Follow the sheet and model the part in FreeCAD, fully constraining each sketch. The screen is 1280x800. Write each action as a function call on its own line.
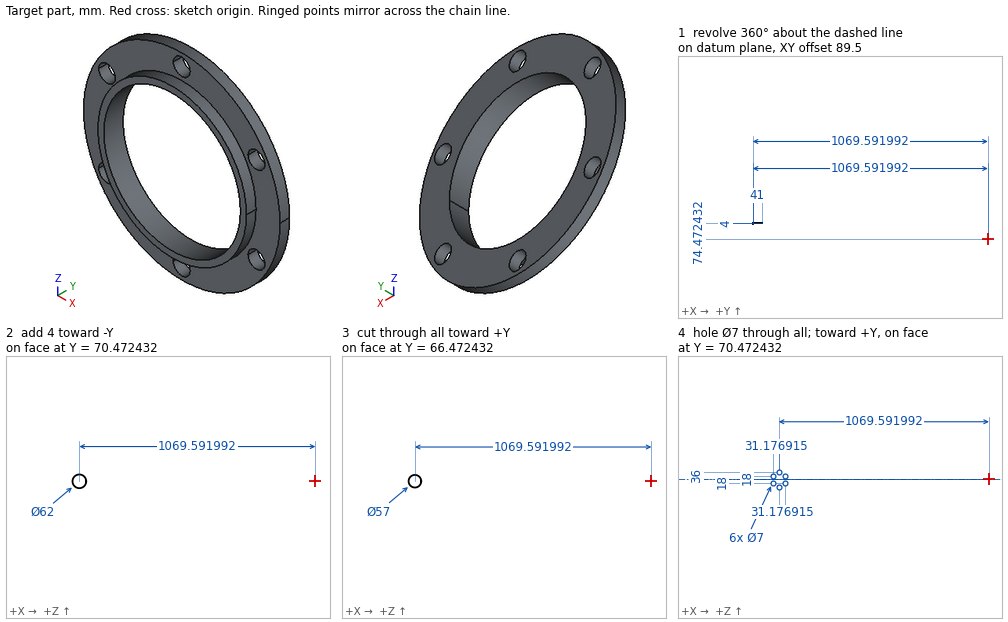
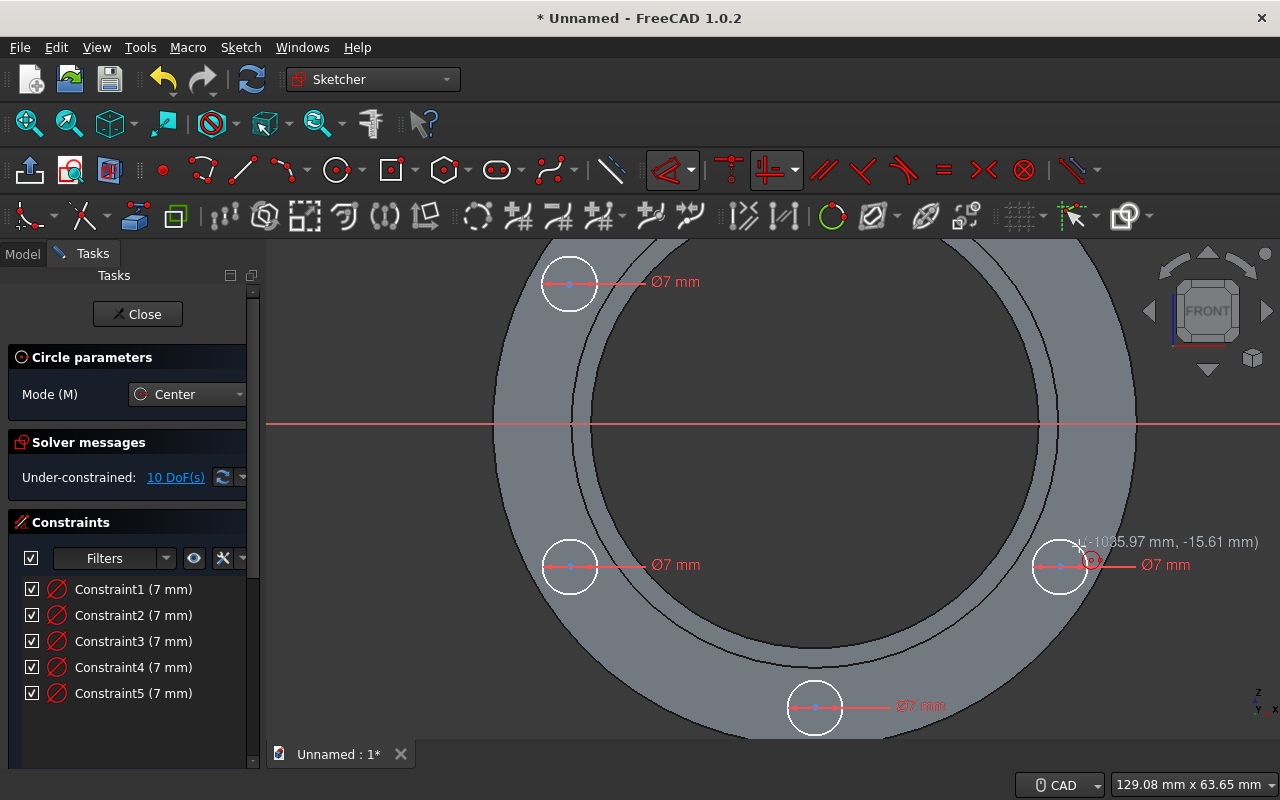
click(1060, 283)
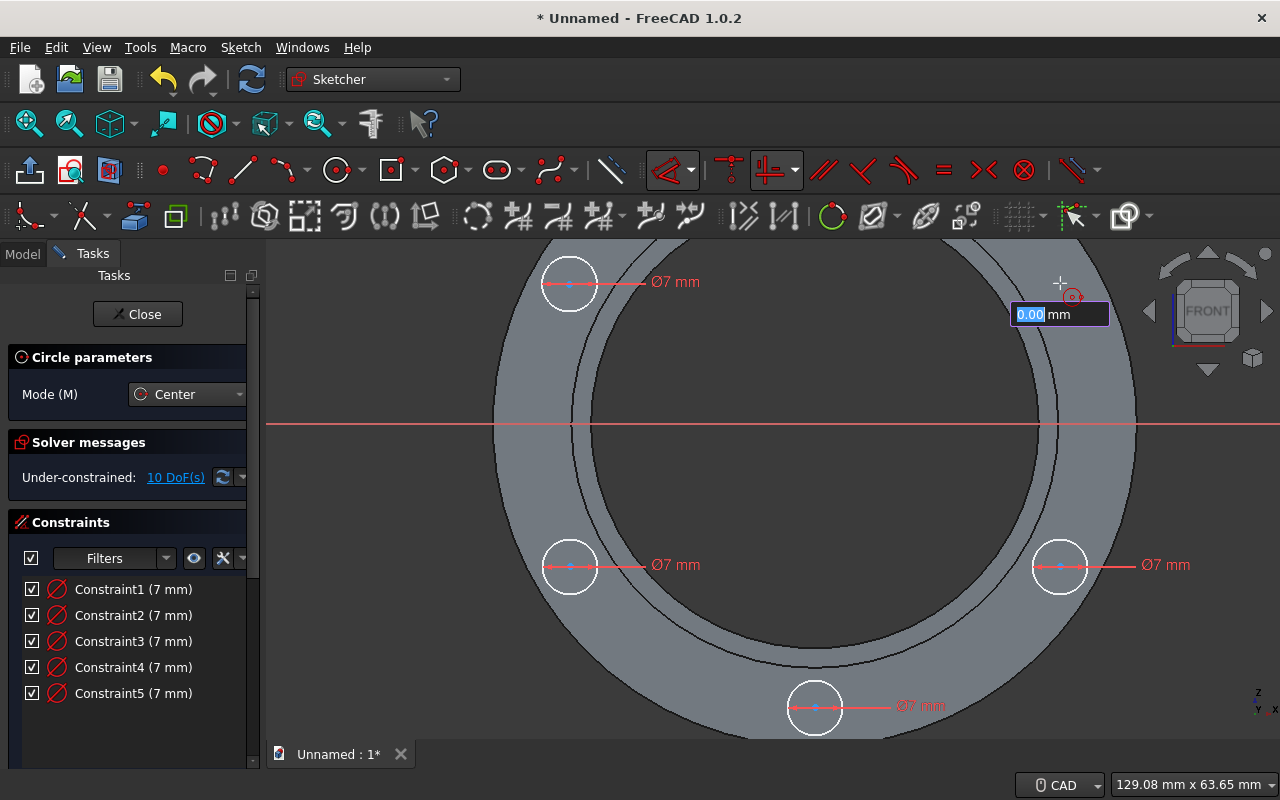
scroll(570, 568, down, 3)
move(850, 401)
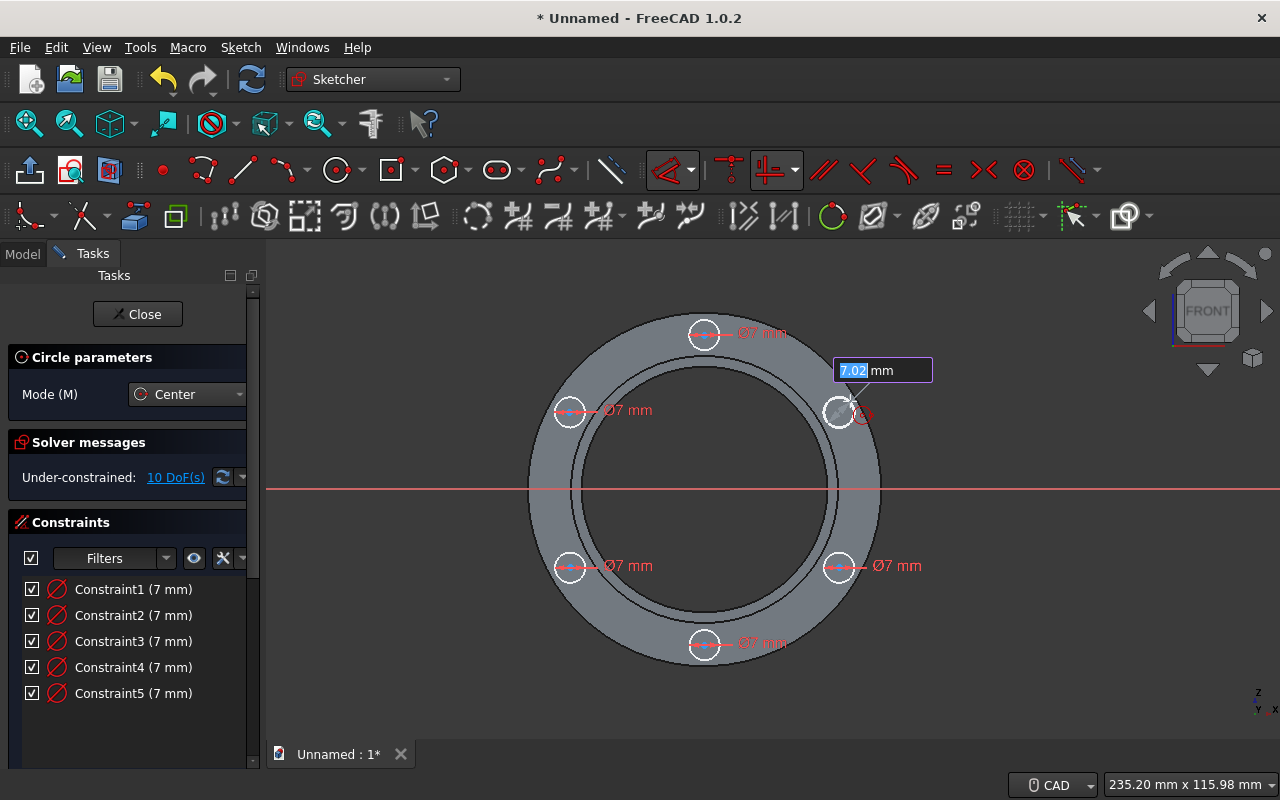
text(7)
key(Return)
key(Escape)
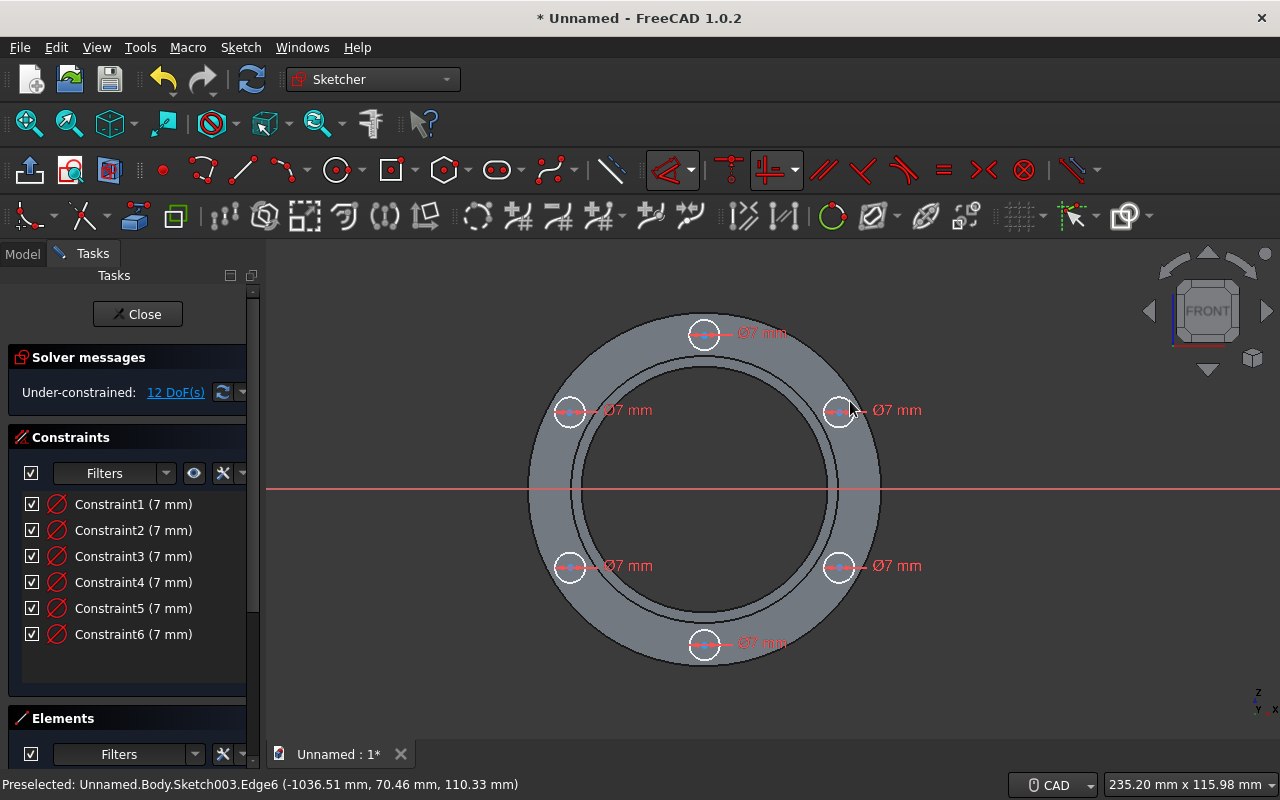
click(570, 412)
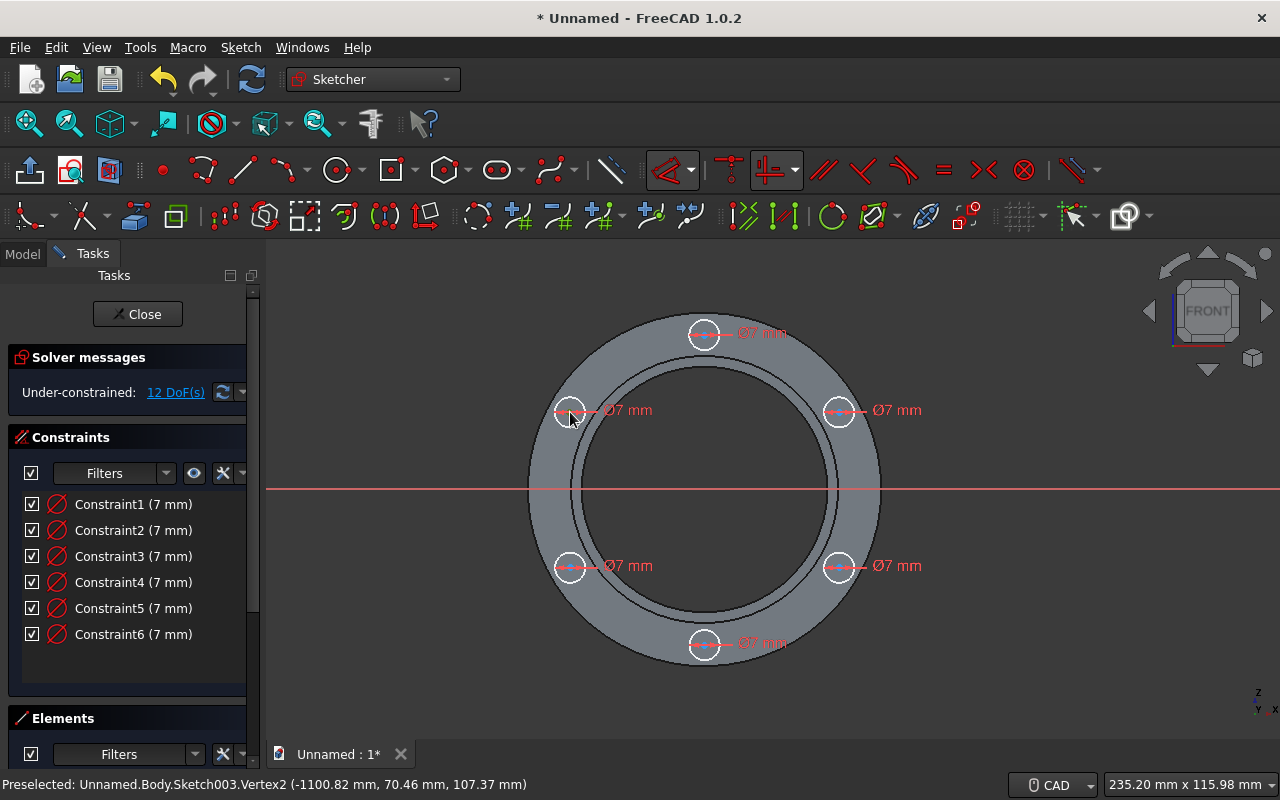
click(570, 568)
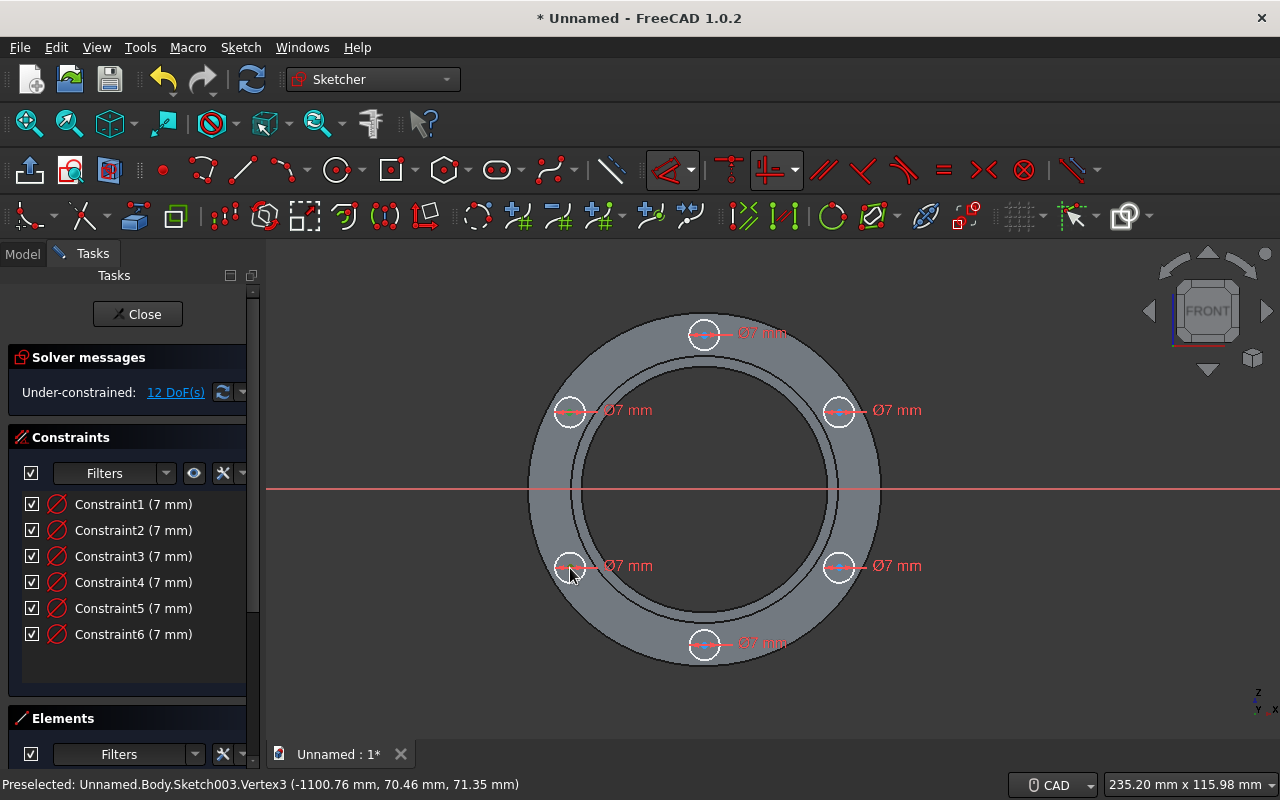
click(353, 489)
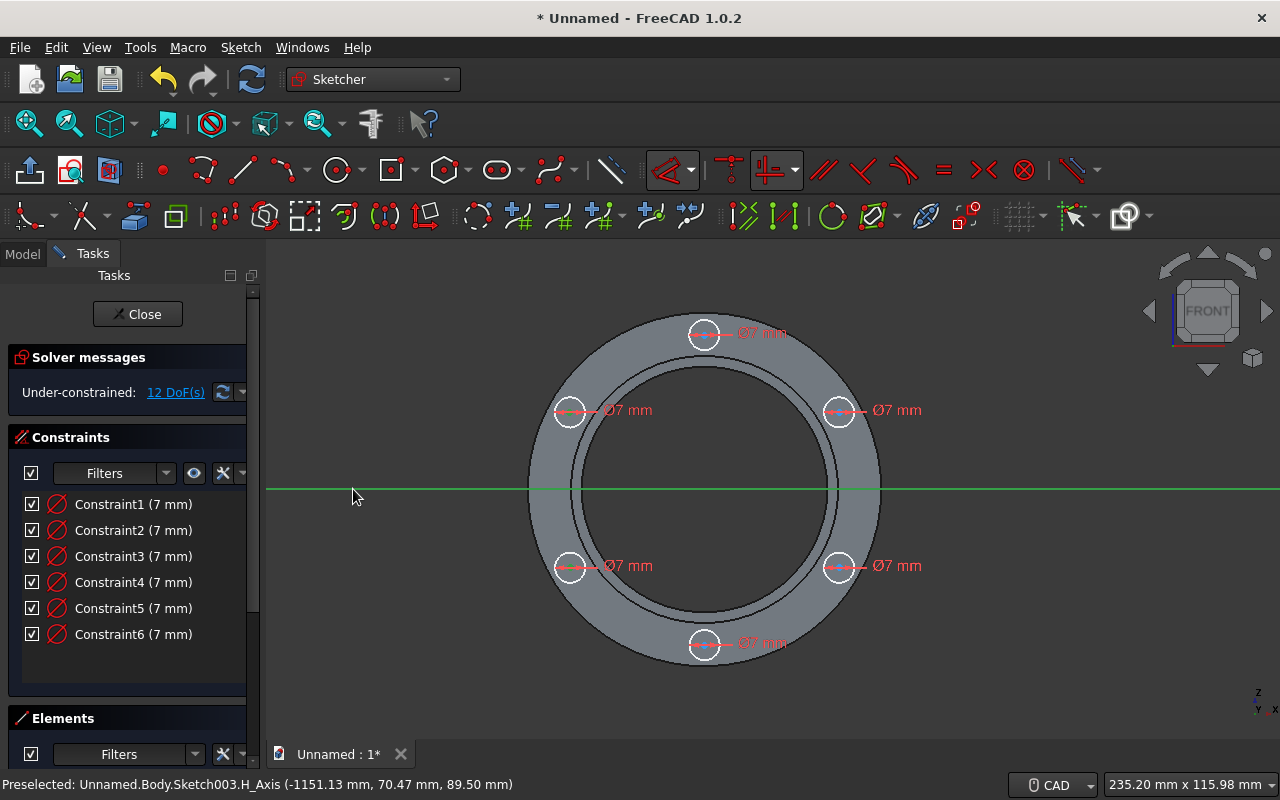
click(984, 170)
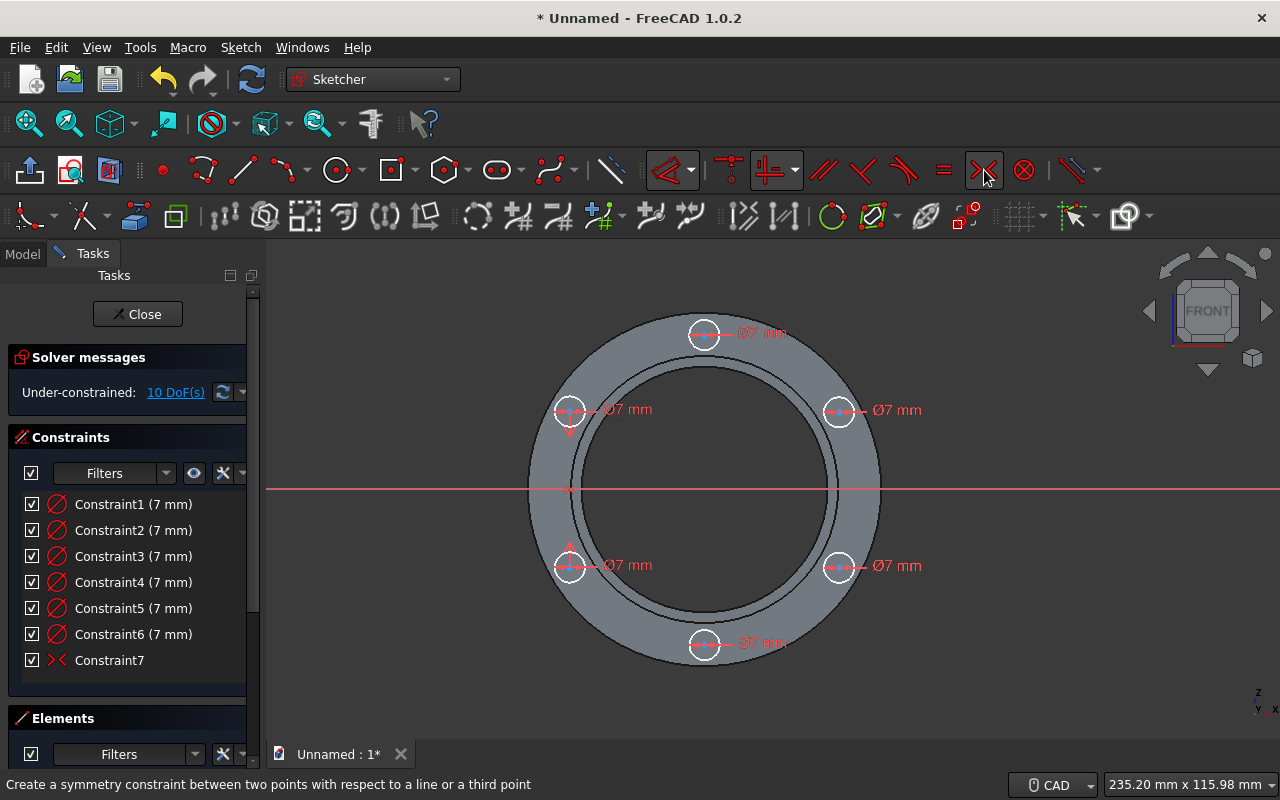
click(704, 335)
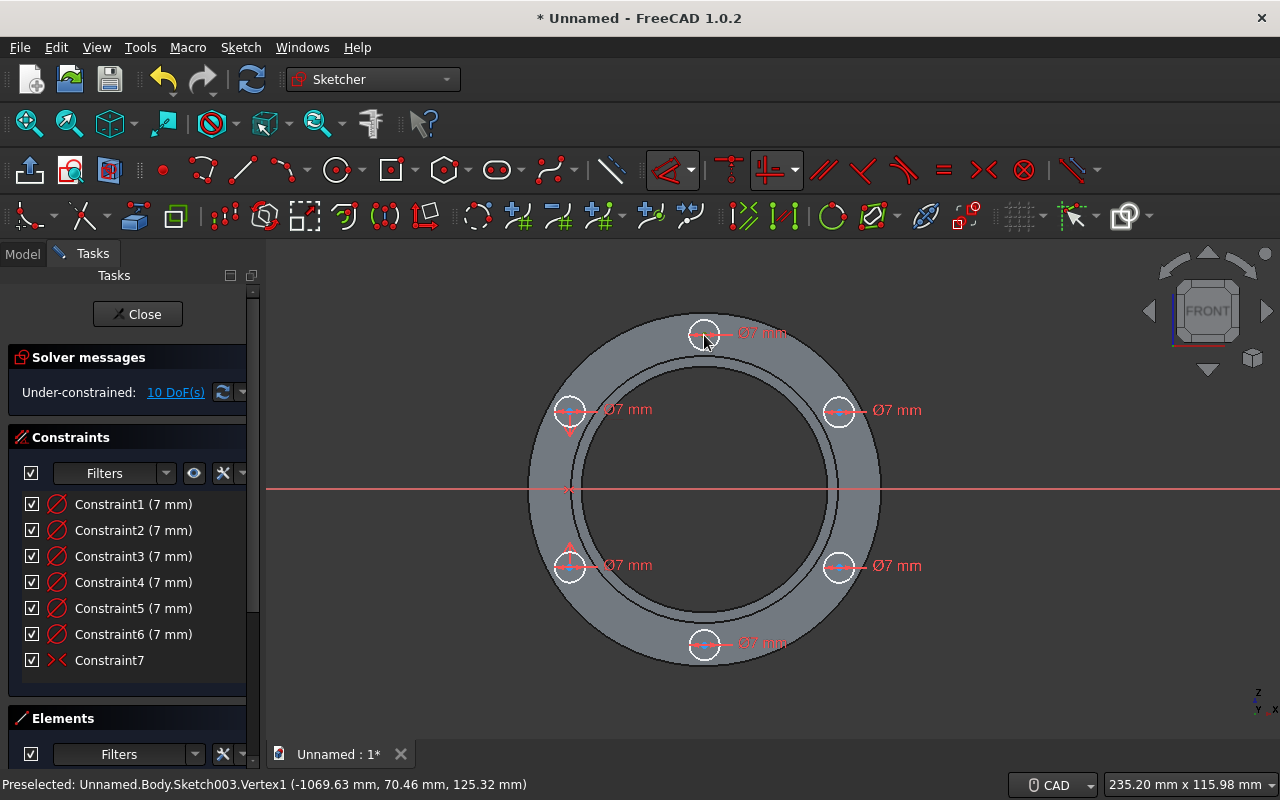
click(705, 645)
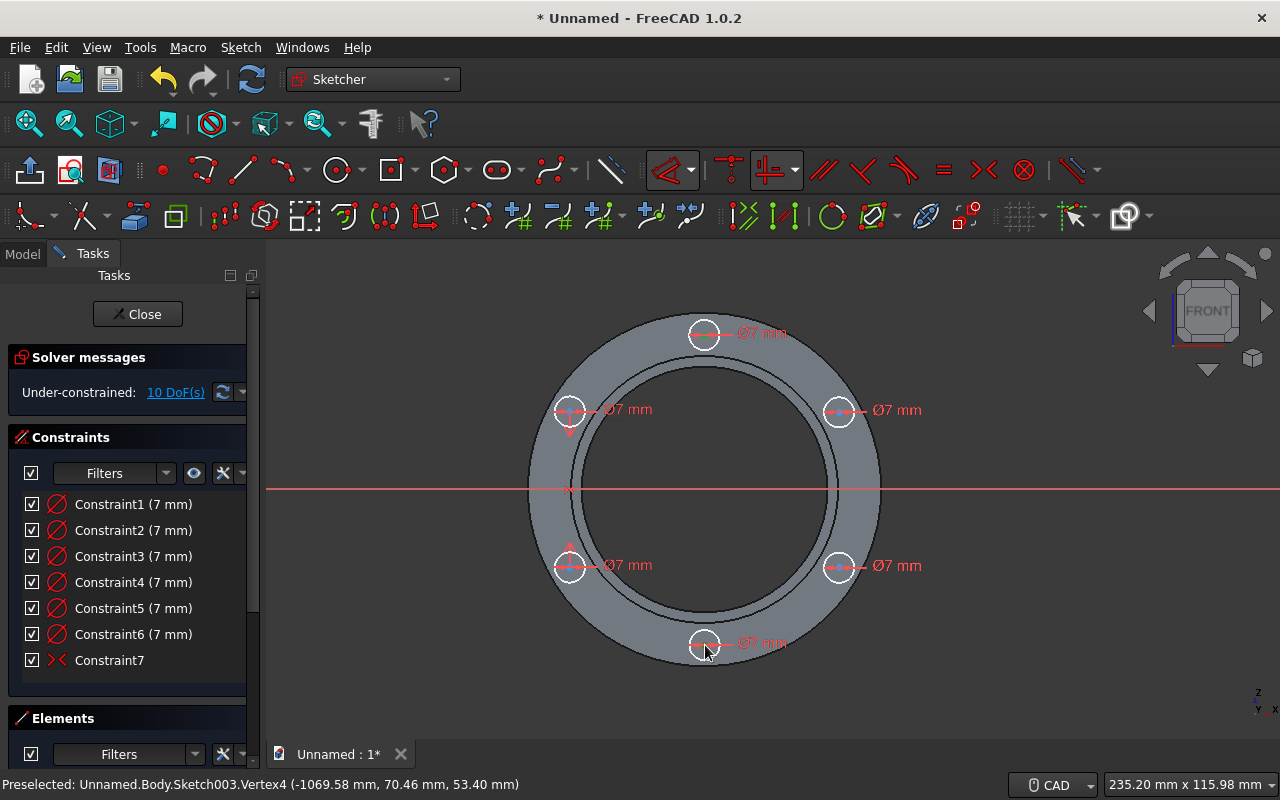
click(353, 489)